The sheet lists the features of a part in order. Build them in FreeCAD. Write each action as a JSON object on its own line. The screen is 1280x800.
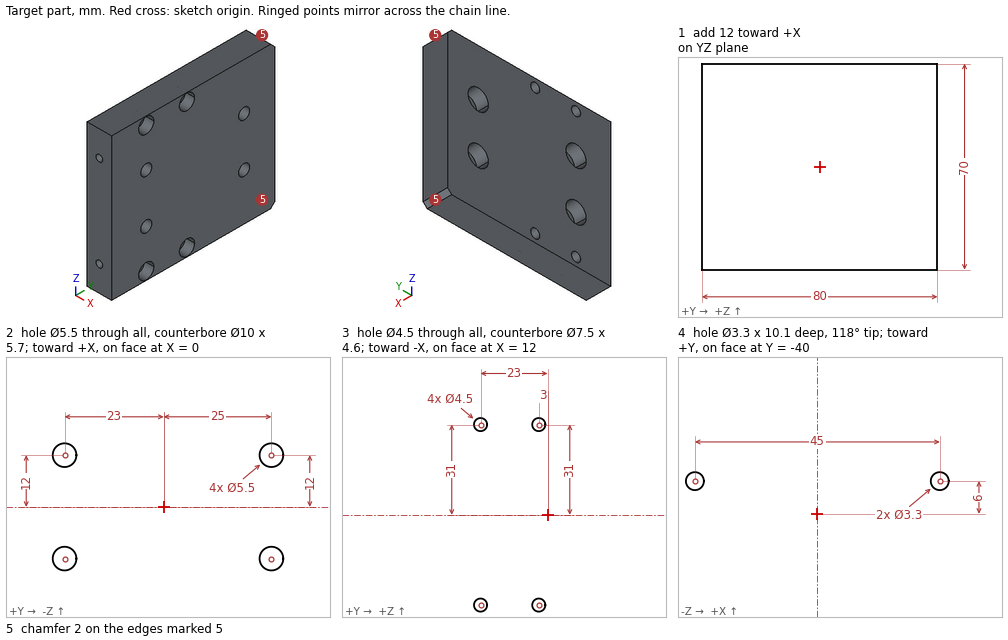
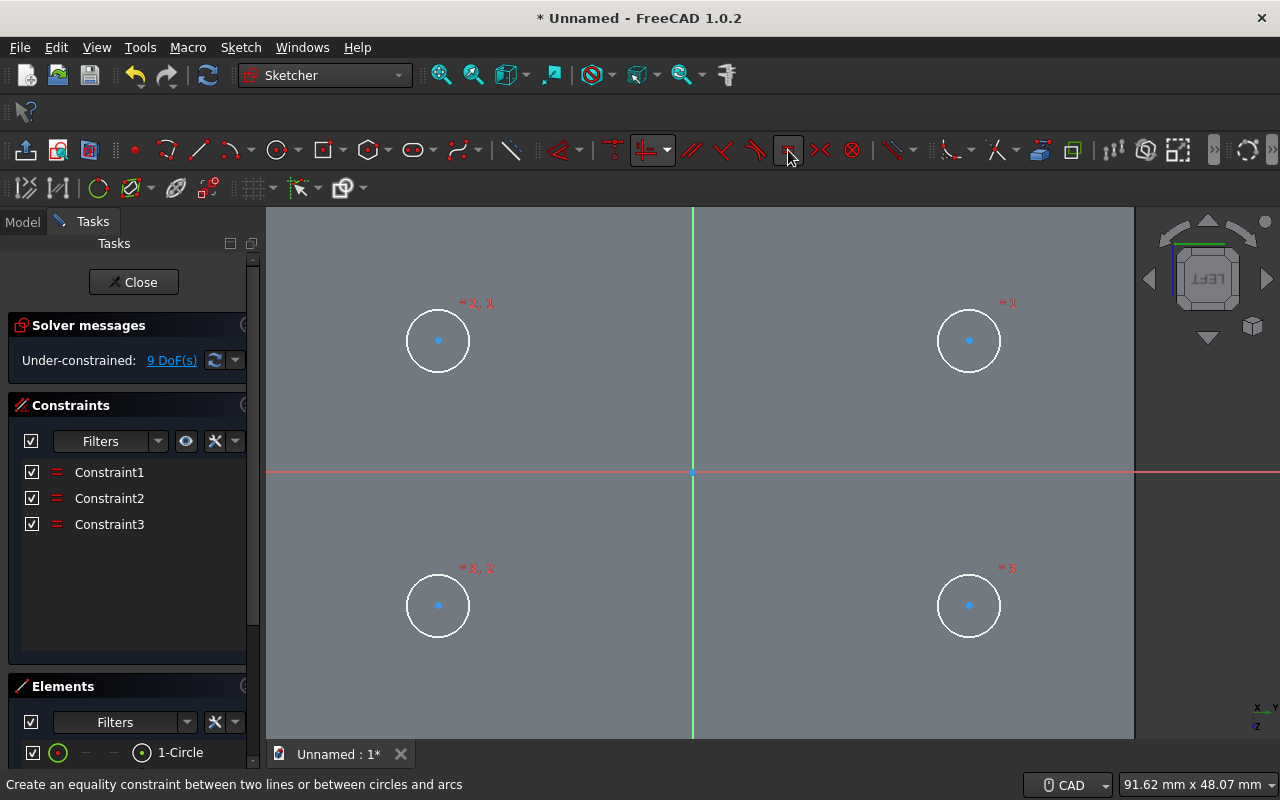
{"action": "left_click", "coordinate": [438, 341]}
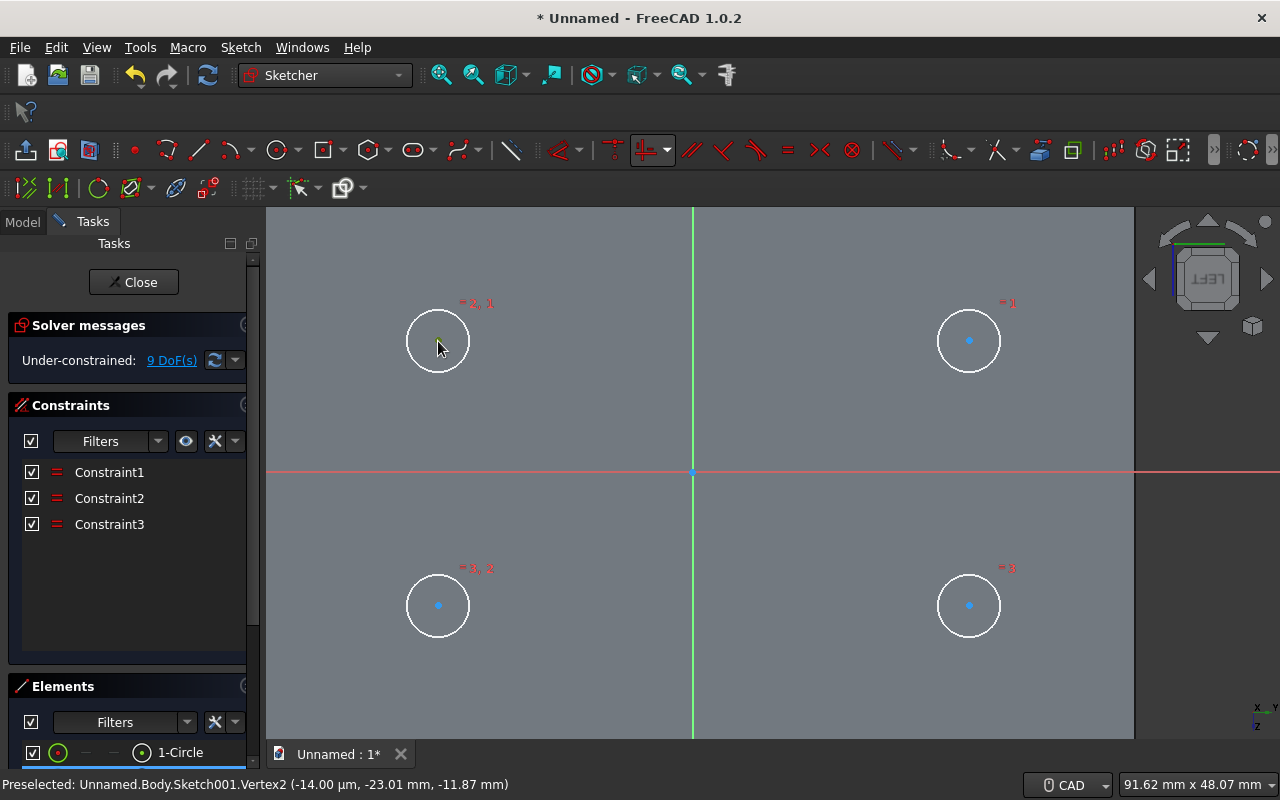
{"action": "left_click", "coordinate": [438, 606]}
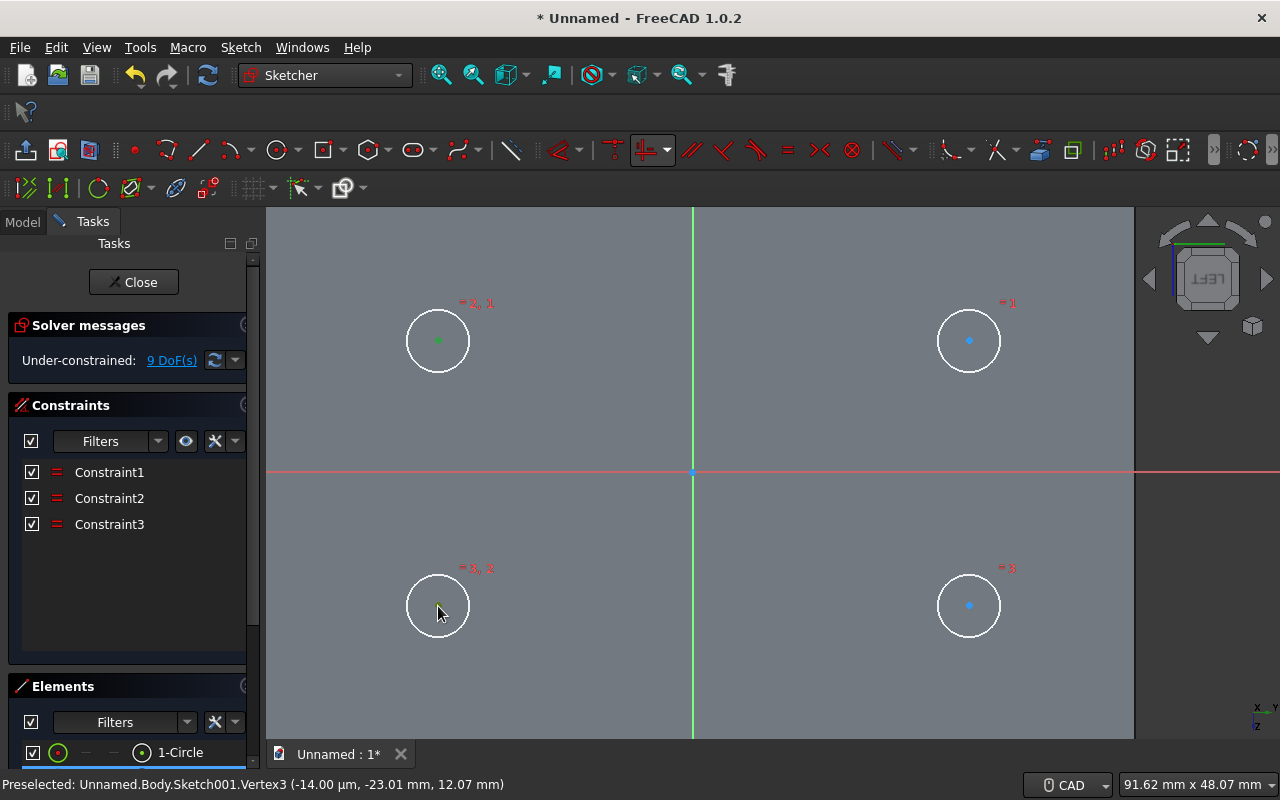
{"action": "left_click", "coordinate": [353, 472]}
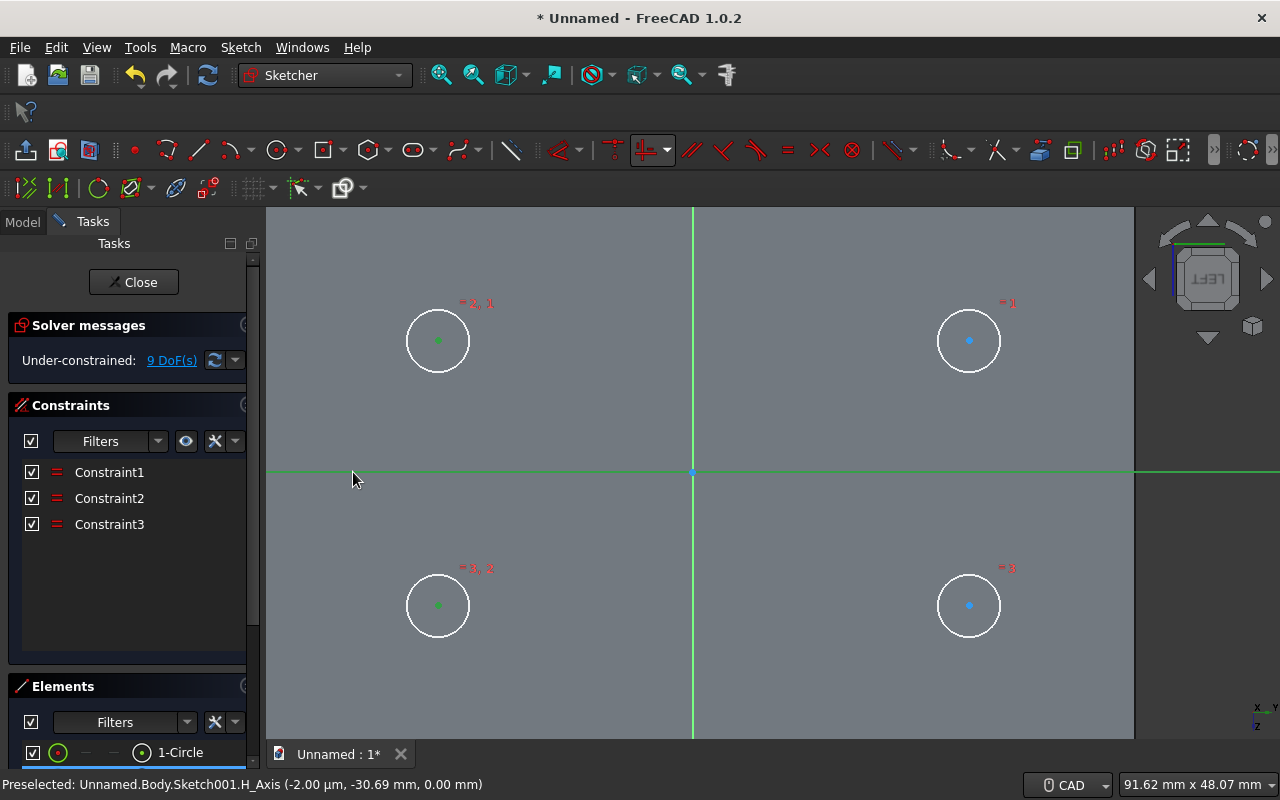
{"action": "left_click", "coordinate": [820, 150]}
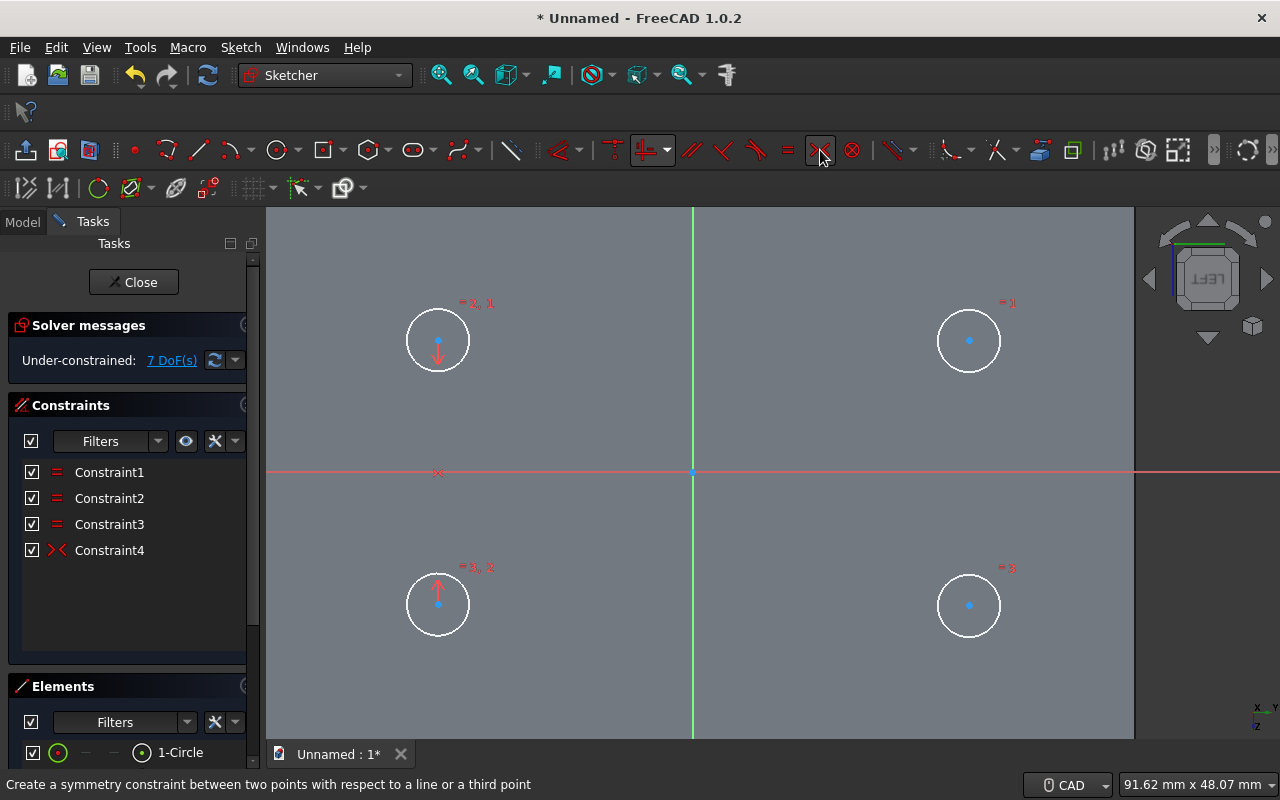
{"action": "left_click", "coordinate": [969, 341]}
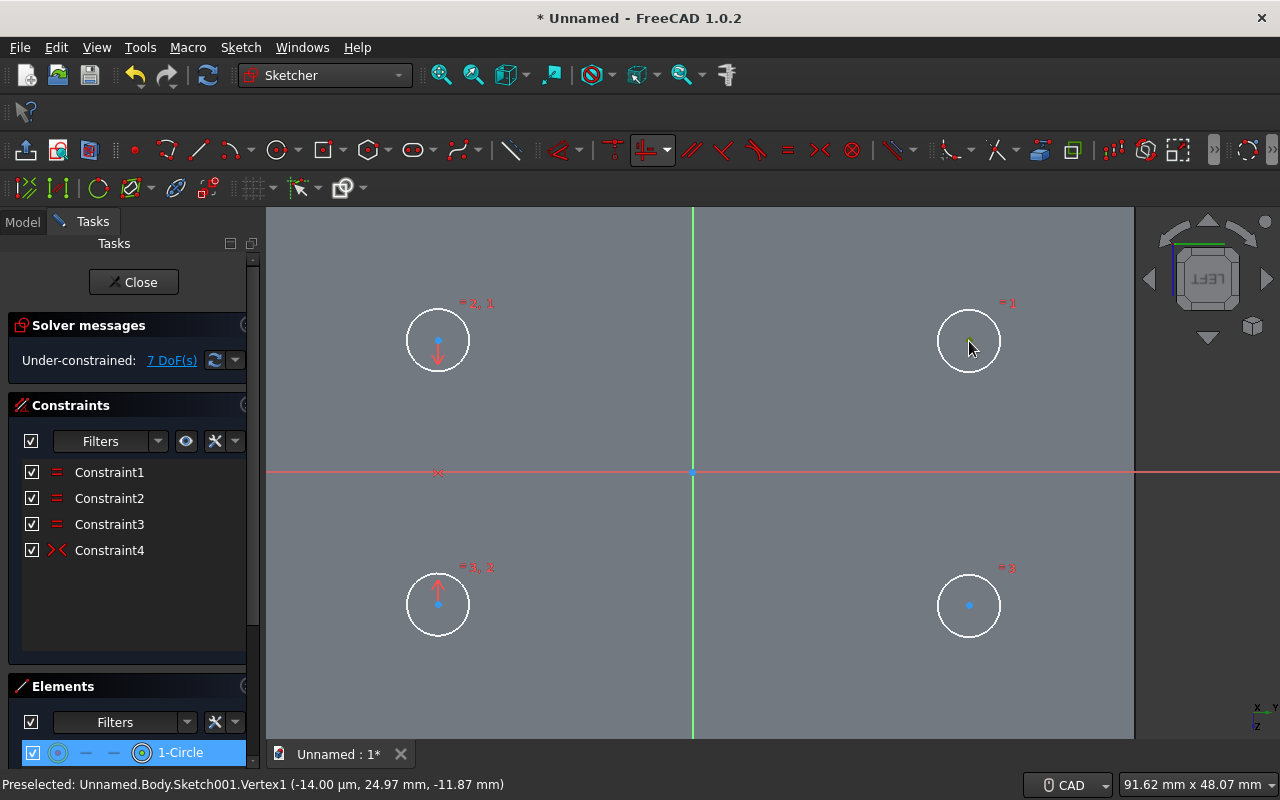
{"action": "left_click", "coordinate": [969, 606]}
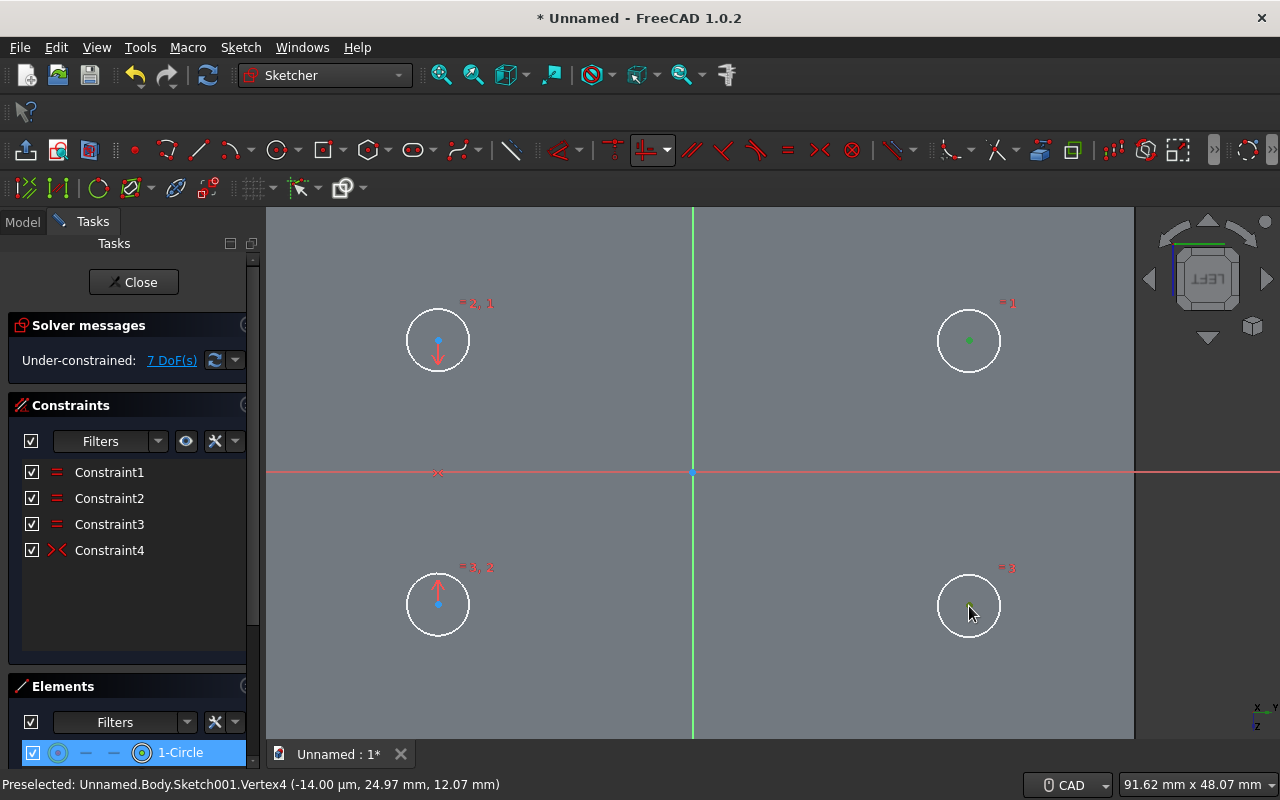
{"action": "left_click", "coordinate": [353, 472]}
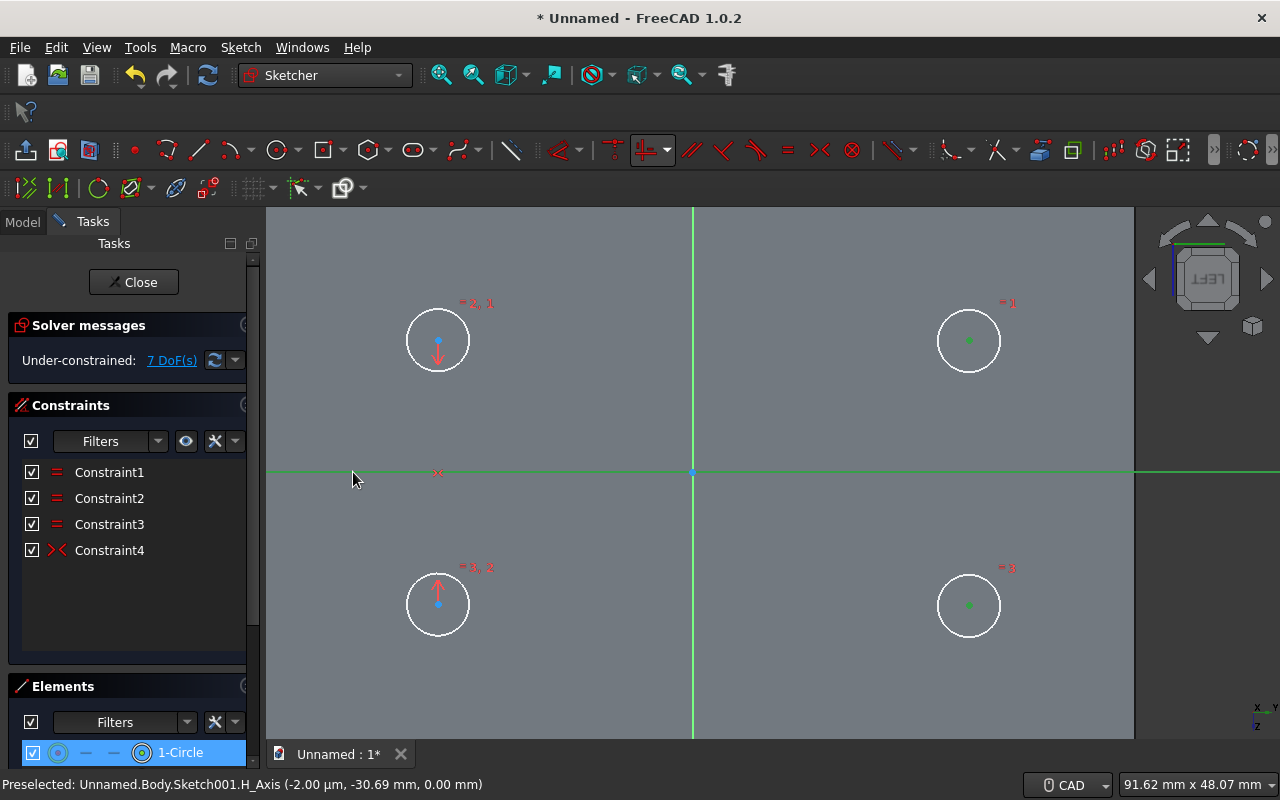
{"action": "left_click", "coordinate": [820, 150]}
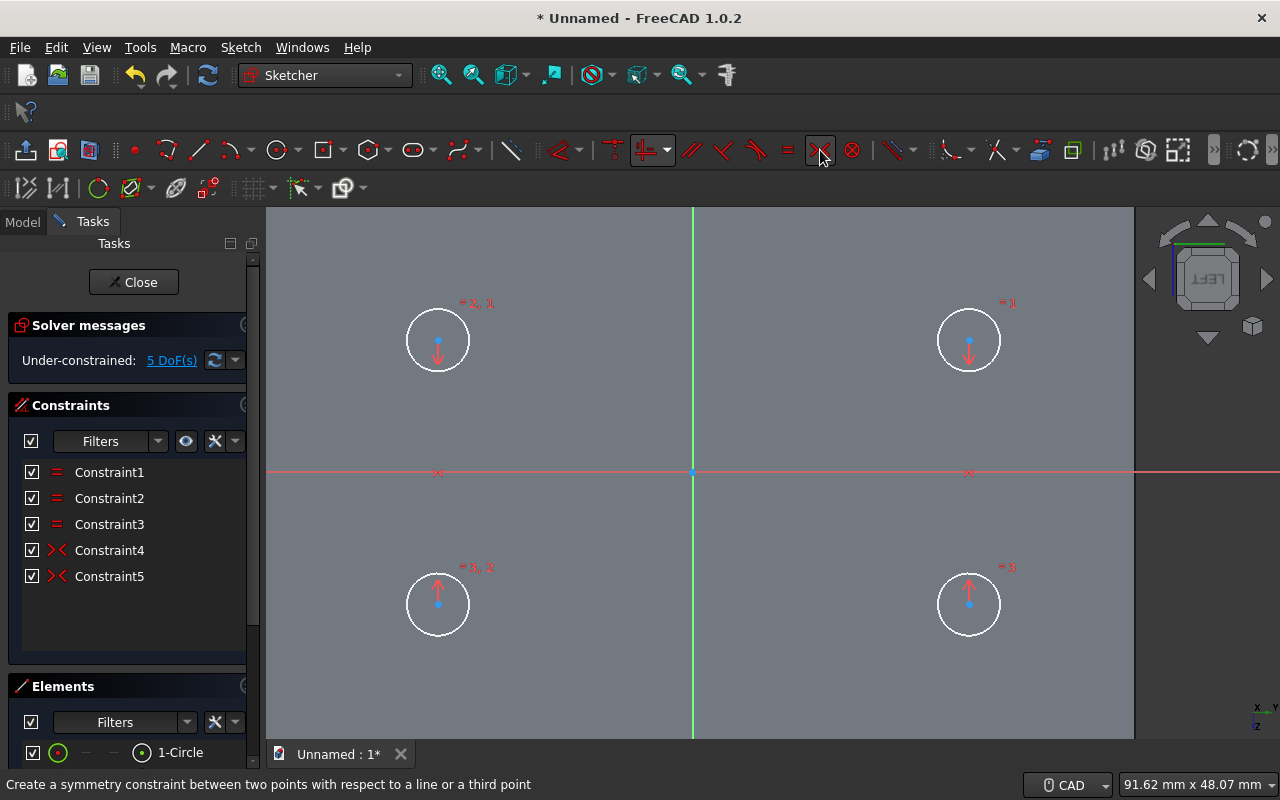
{"action": "left_click", "coordinate": [558, 150]}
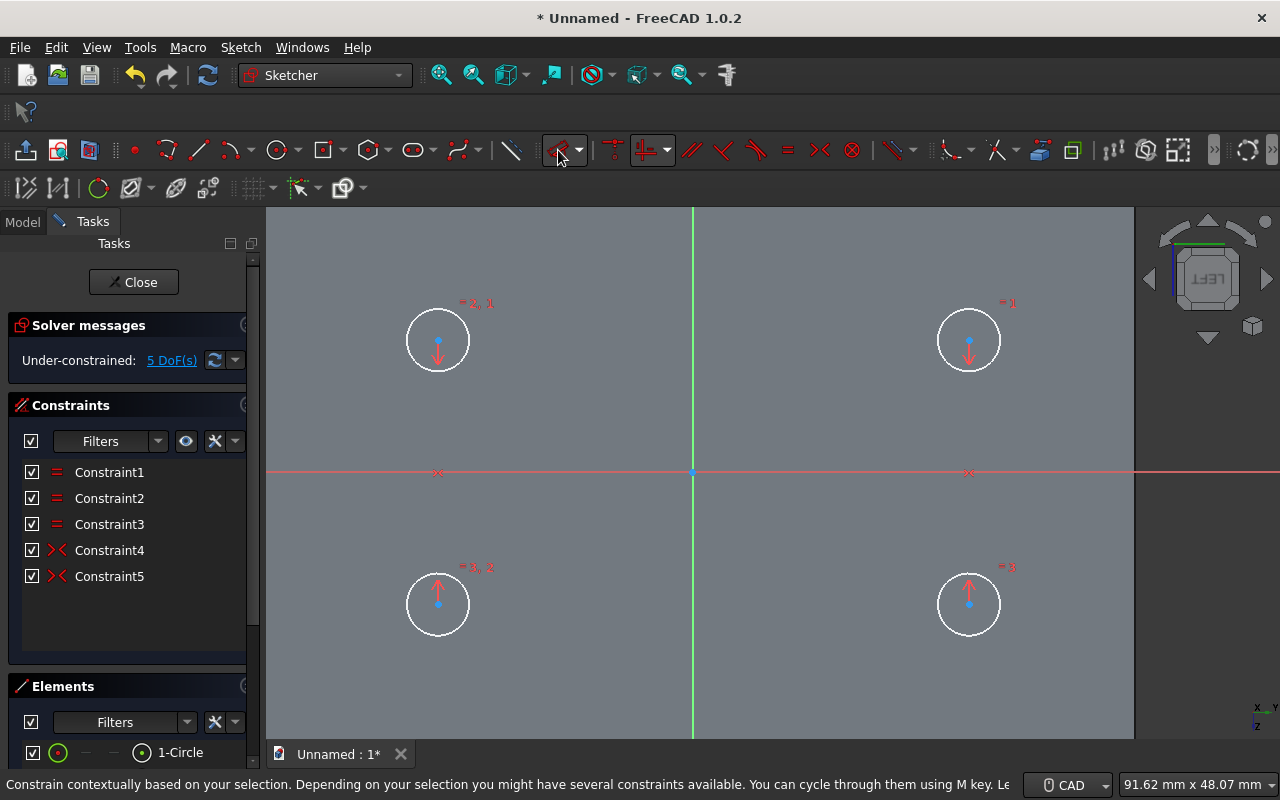
{"action": "left_click", "coordinate": [991, 318]}
{"action": "left_click", "coordinate": [1014, 295]}